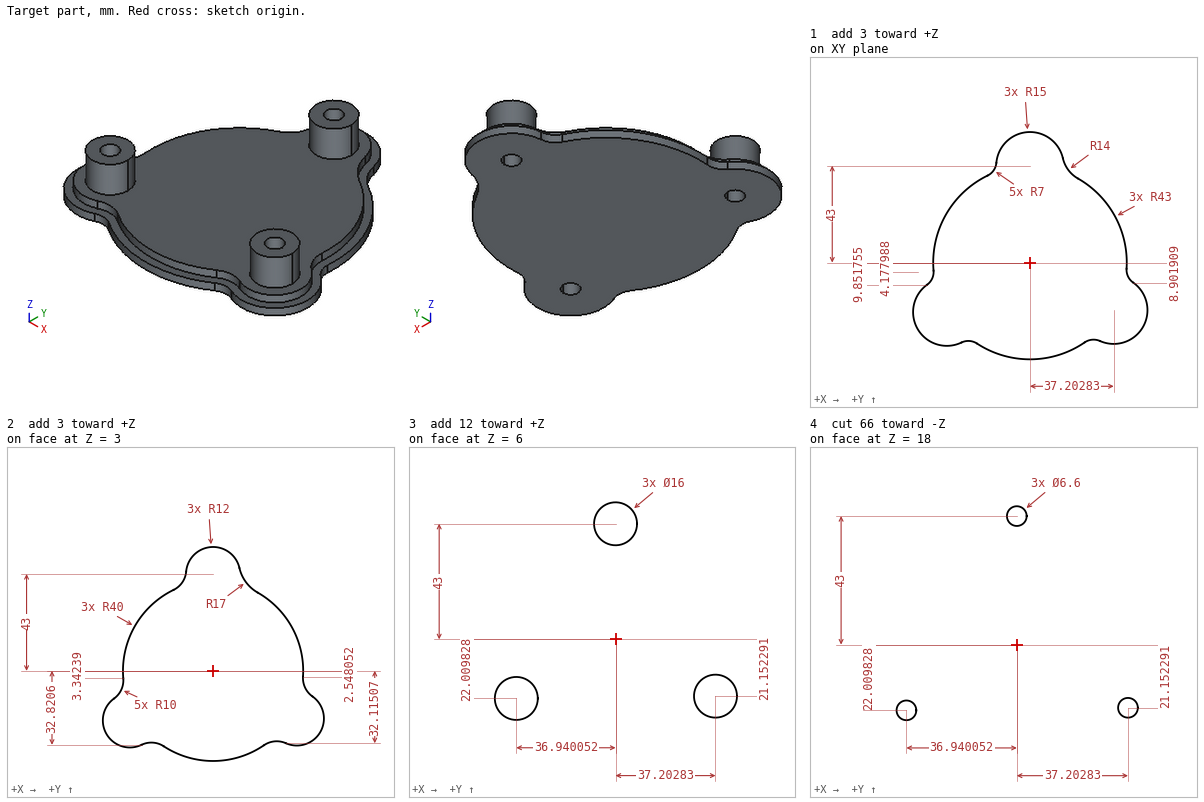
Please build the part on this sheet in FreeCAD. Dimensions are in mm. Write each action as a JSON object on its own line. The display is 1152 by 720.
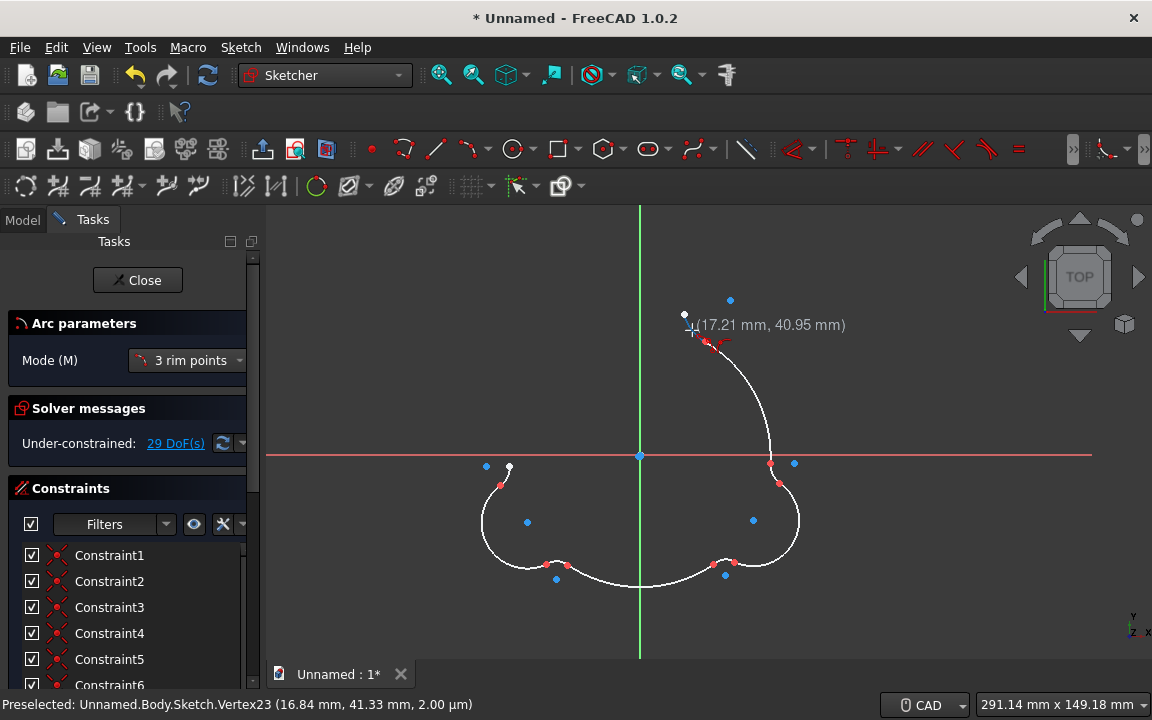
{"action": "left_click", "coordinate": [684, 315]}
{"action": "left_click", "coordinate": [595, 320]}
{"action": "left_click", "coordinate": [624, 281]}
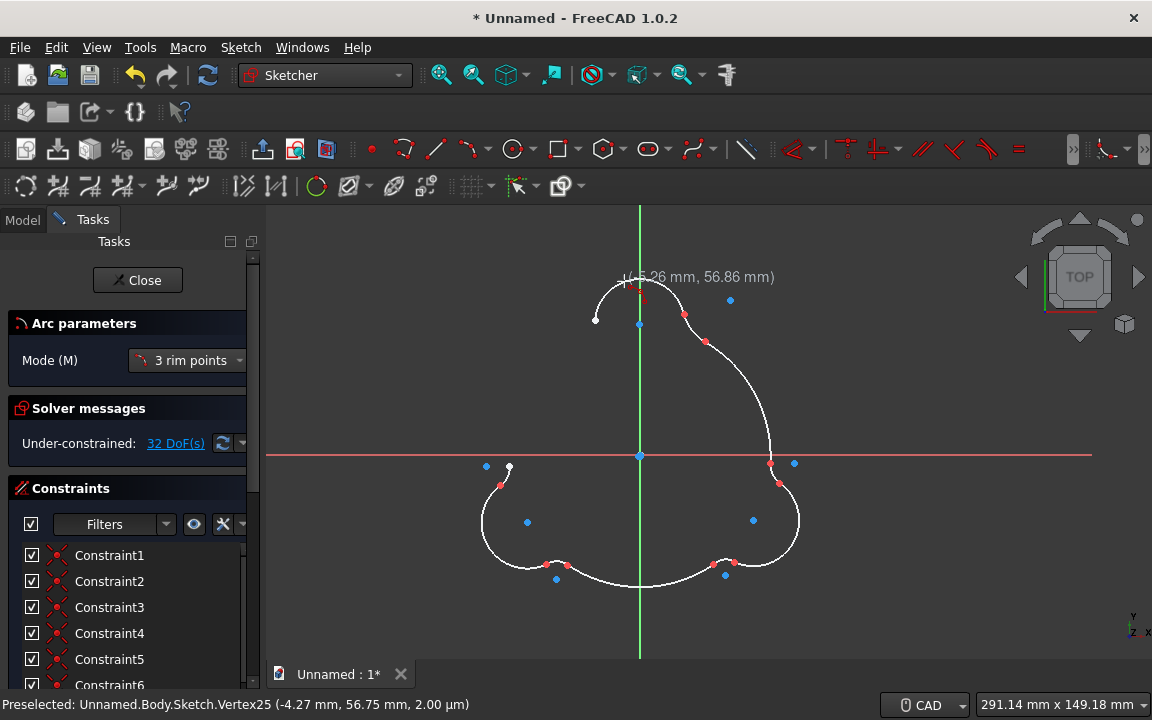
{"action": "left_click", "coordinate": [595, 321]}
{"action": "left_click", "coordinate": [583, 337]}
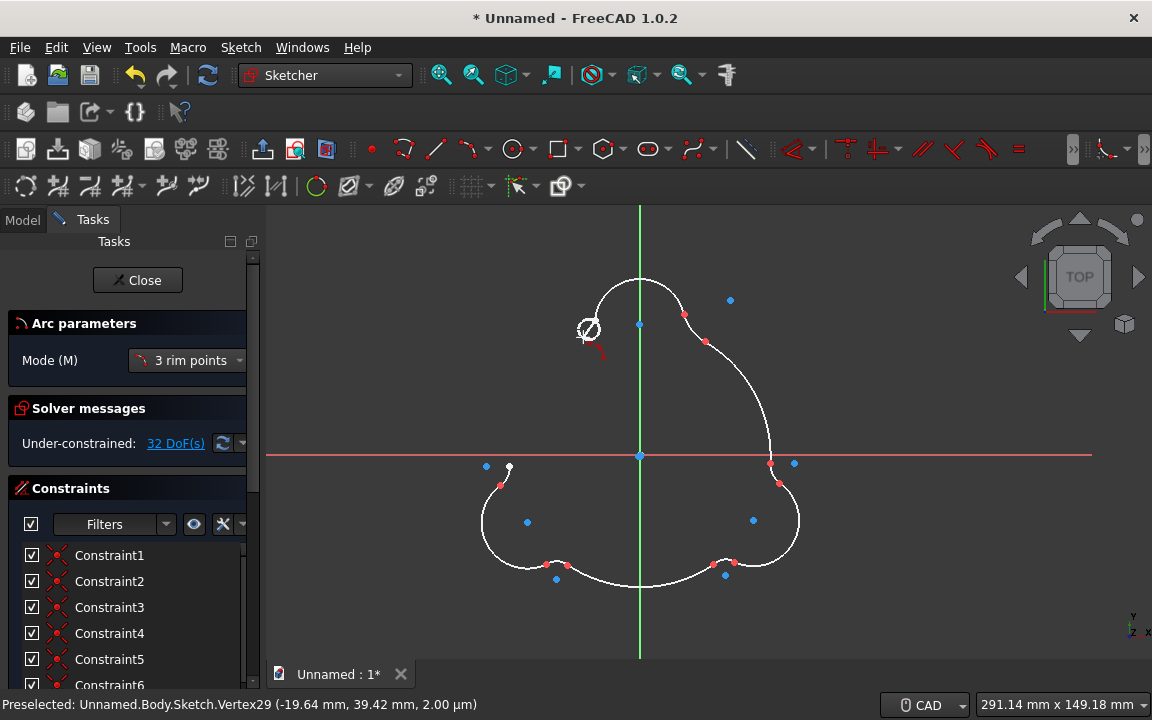
{"action": "scroll", "coordinate": [591, 330], "scroll_direction": "up", "scroll_amount": 9}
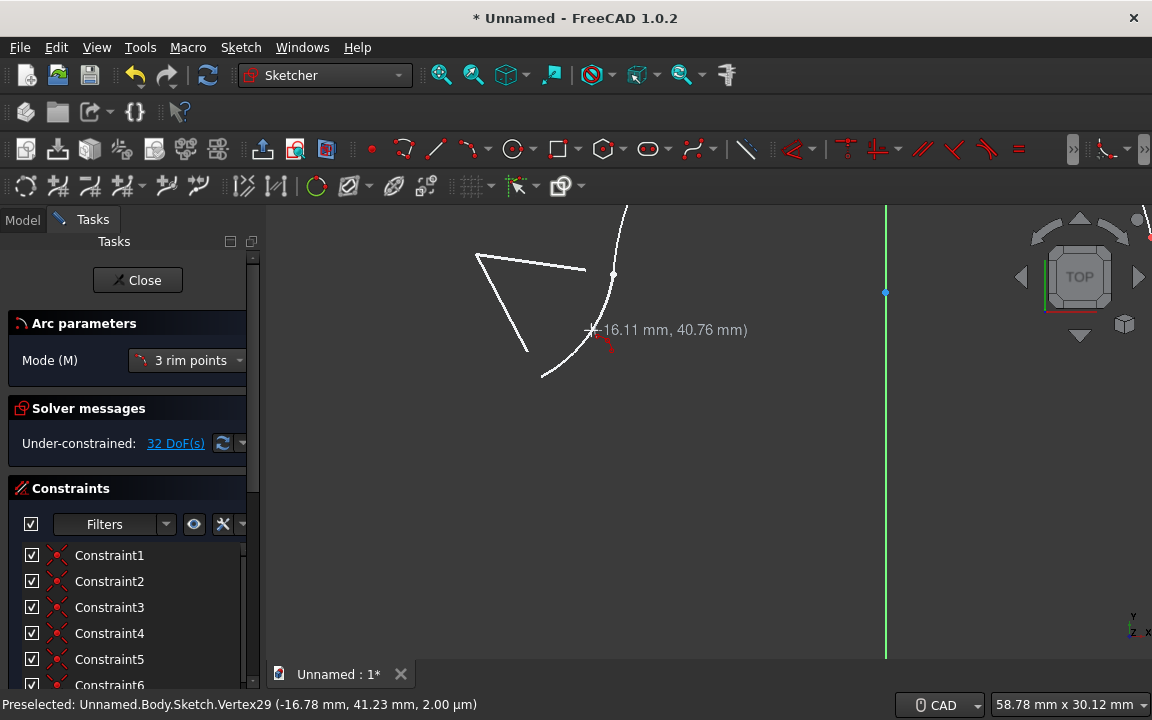
{"action": "left_click", "coordinate": [588, 331]}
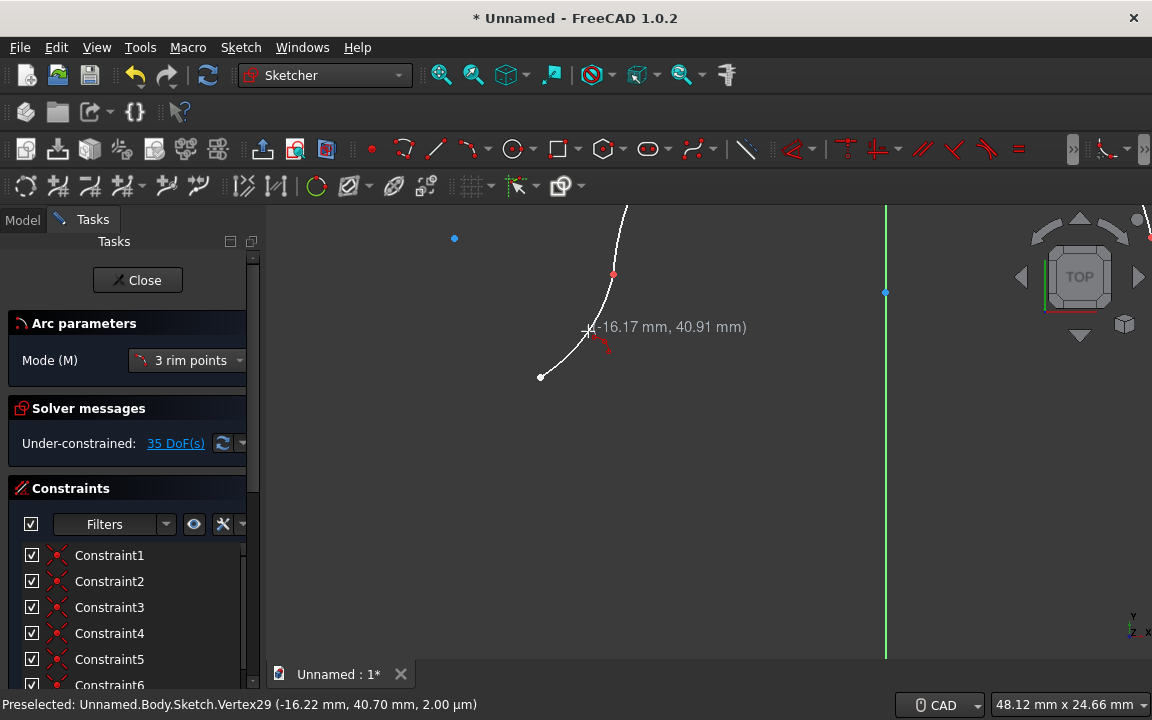
{"action": "scroll", "coordinate": [591, 330], "scroll_direction": "down", "scroll_amount": 9}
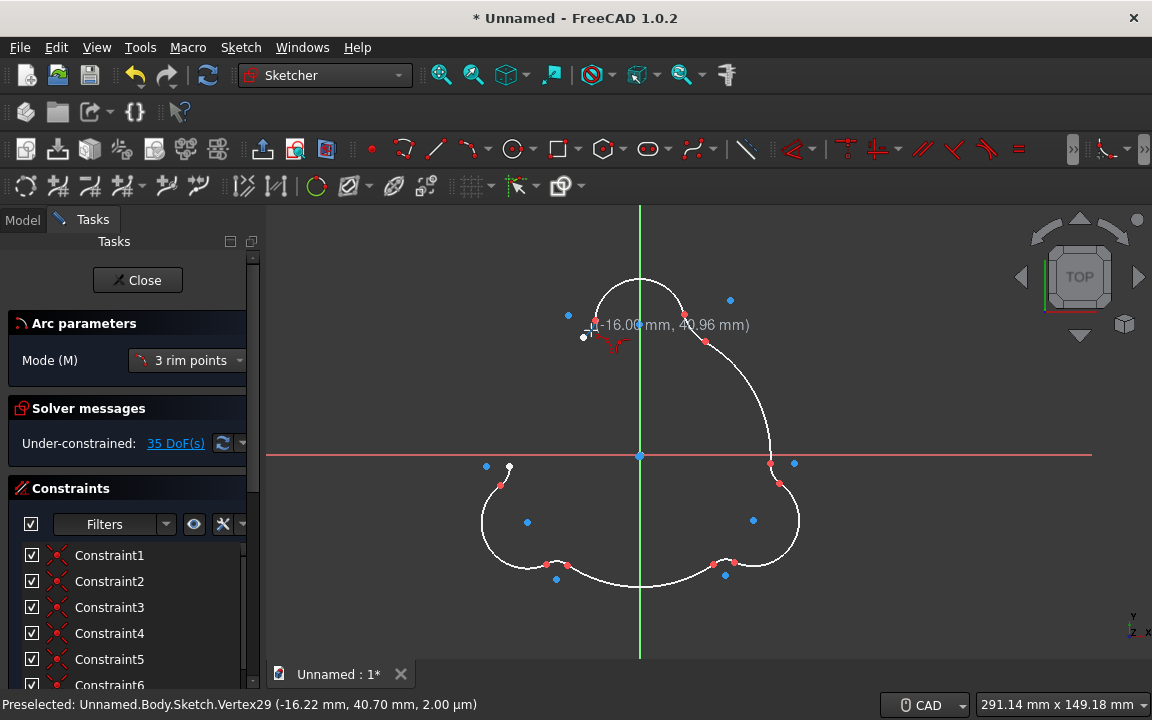
{"action": "left_click", "coordinate": [583, 338]}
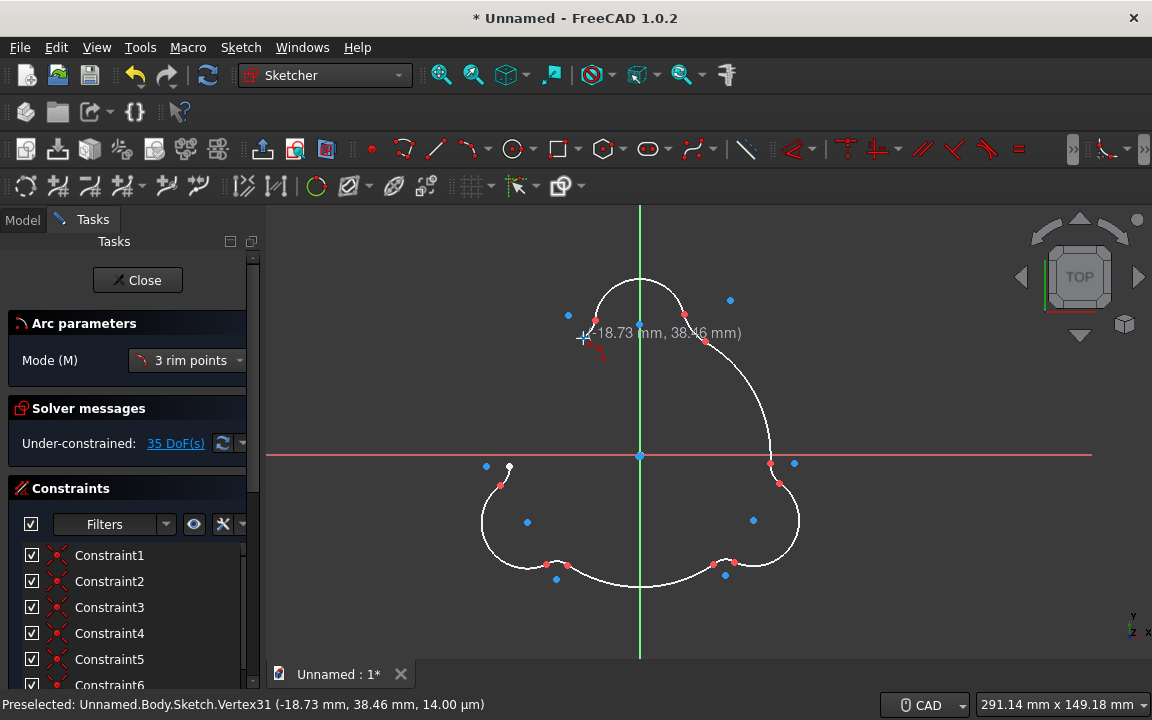
{"action": "scroll", "coordinate": [510, 466], "scroll_direction": "up", "scroll_amount": 2}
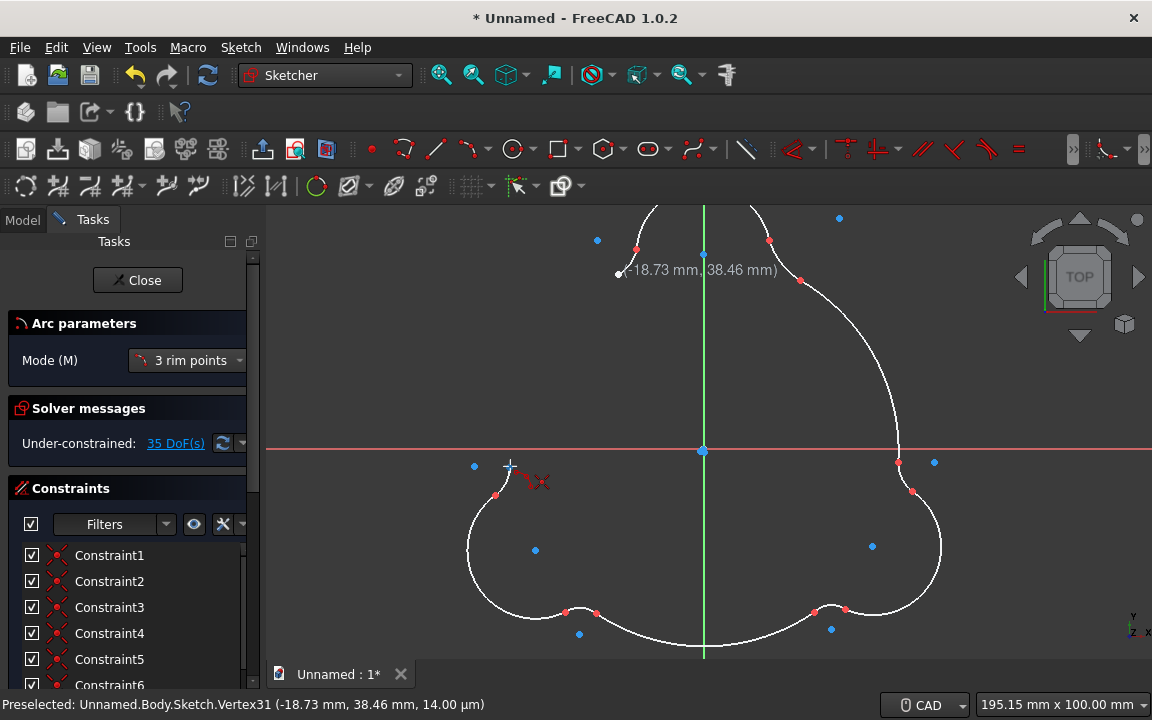
{"action": "left_click", "coordinate": [510, 467]}
{"action": "left_click", "coordinate": [534, 353]}
{"action": "key", "text": "Escape"}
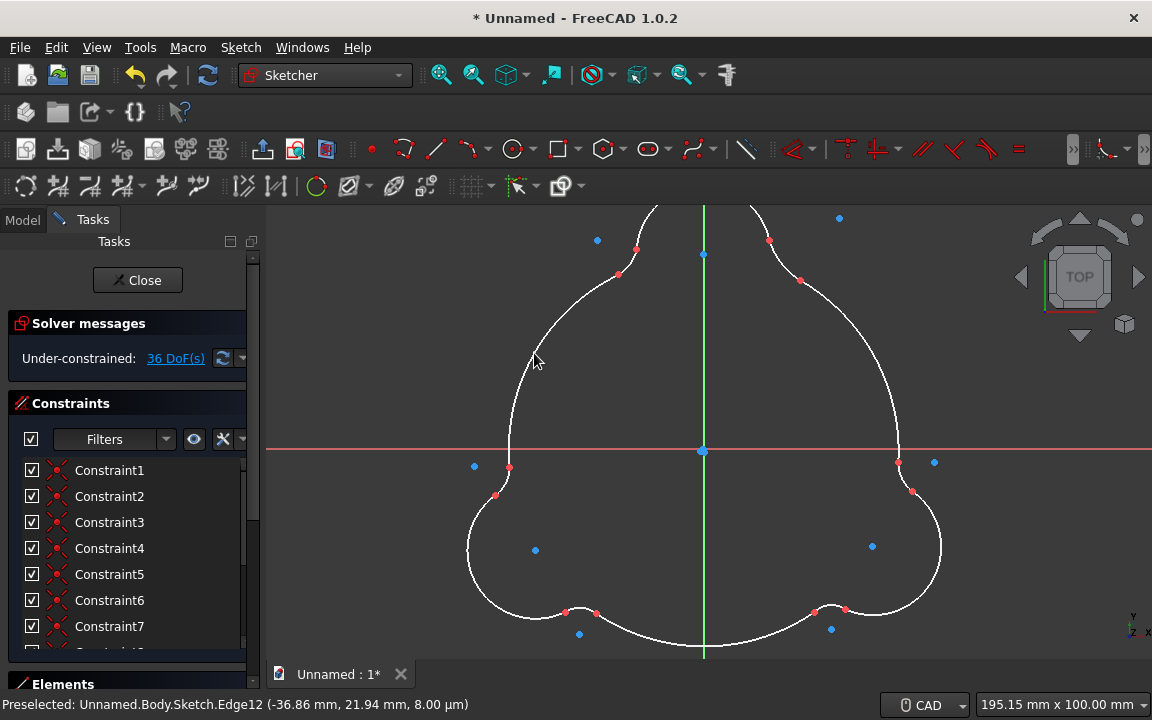
{"action": "scroll", "coordinate": [503, 488], "scroll_direction": "up", "scroll_amount": 2}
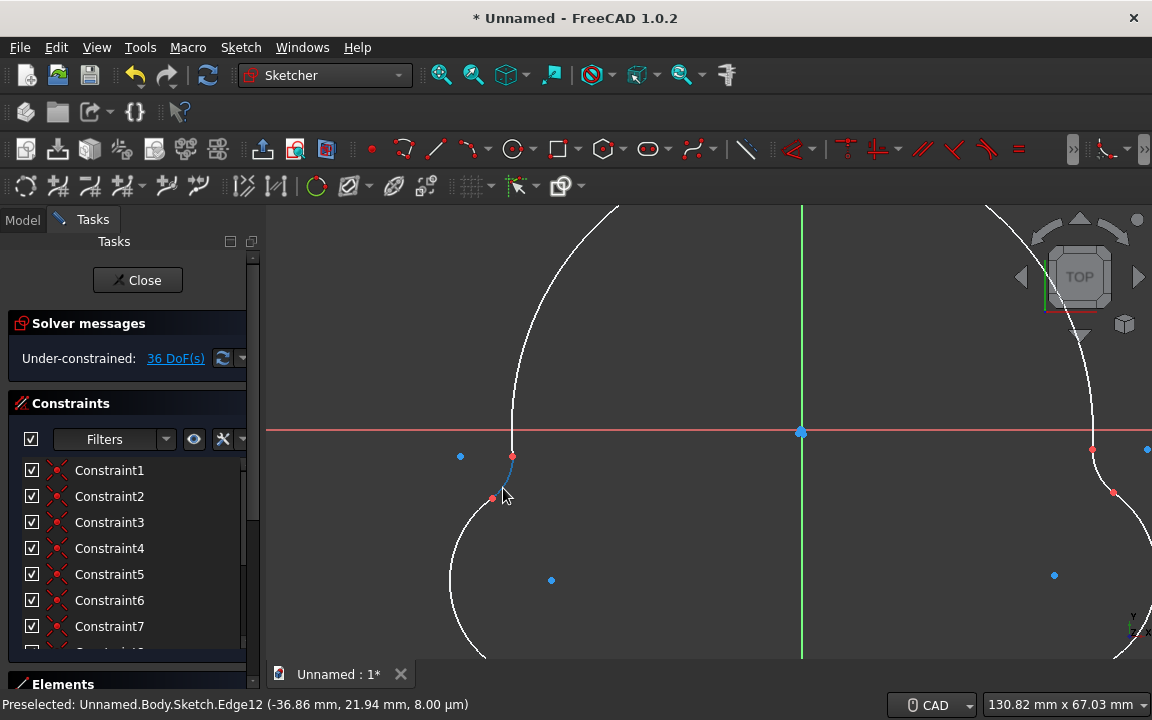
{"action": "left_click", "coordinate": [502, 488]}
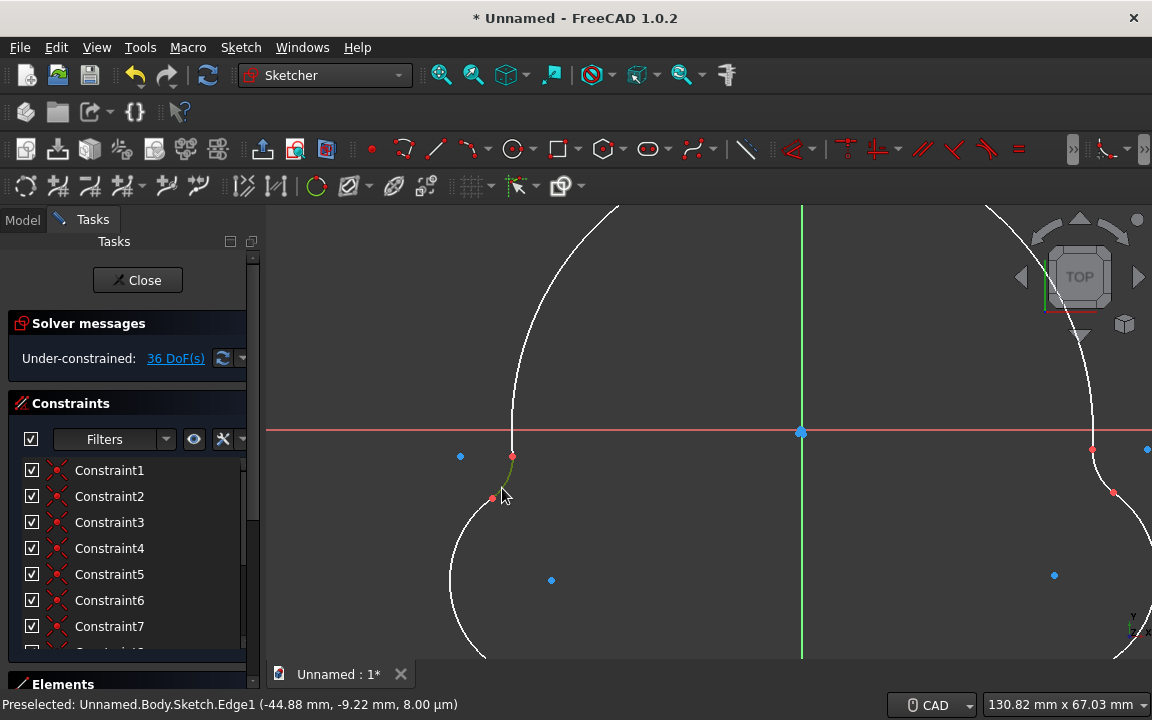
{"action": "left_click", "coordinate": [450, 575]}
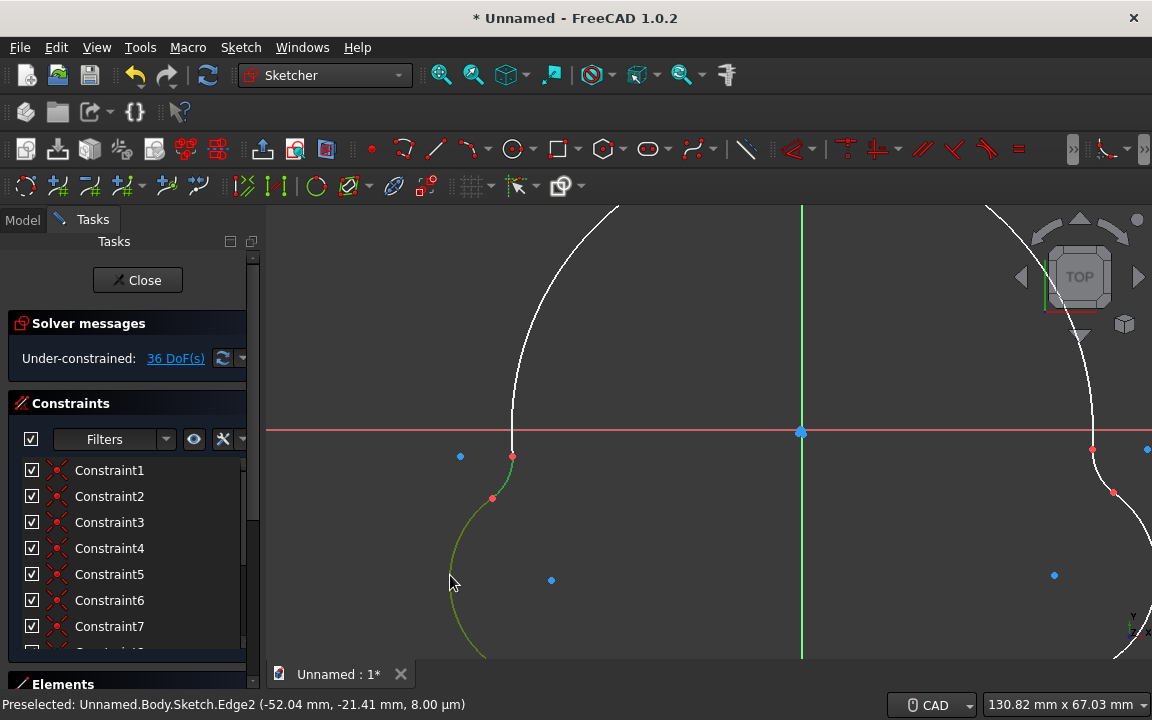
{"action": "left_click", "coordinate": [988, 150]}